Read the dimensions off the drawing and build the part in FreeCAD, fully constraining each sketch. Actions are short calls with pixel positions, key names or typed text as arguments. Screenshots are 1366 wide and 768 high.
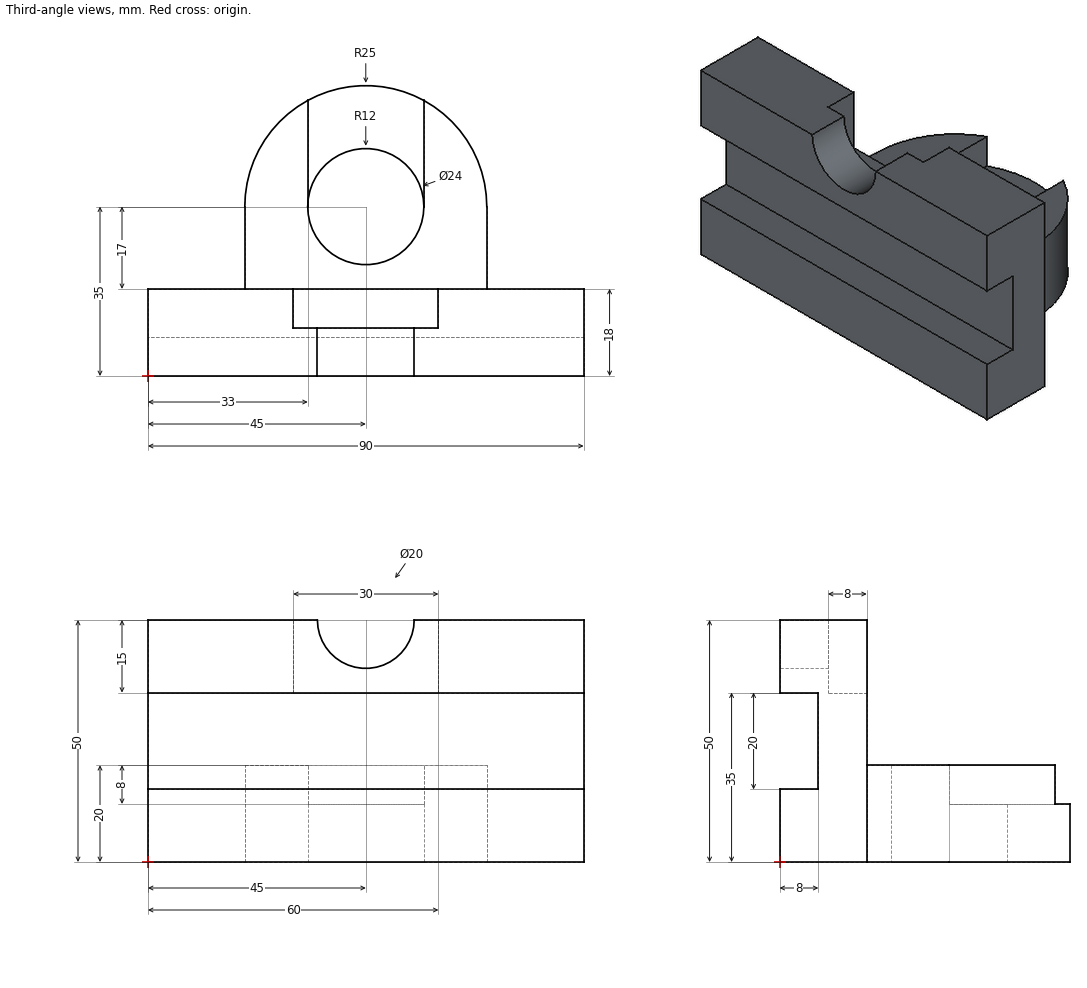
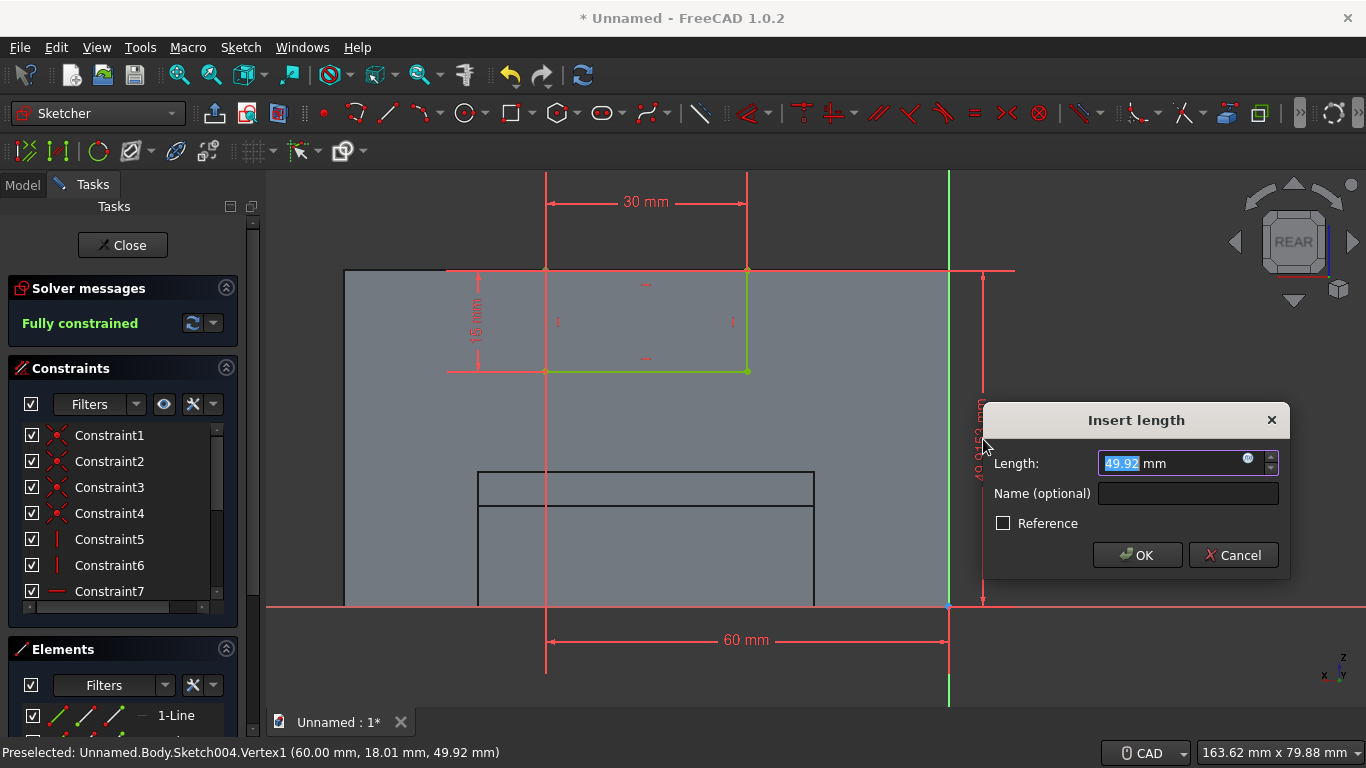
text(50)
key(Return)
key(Escape)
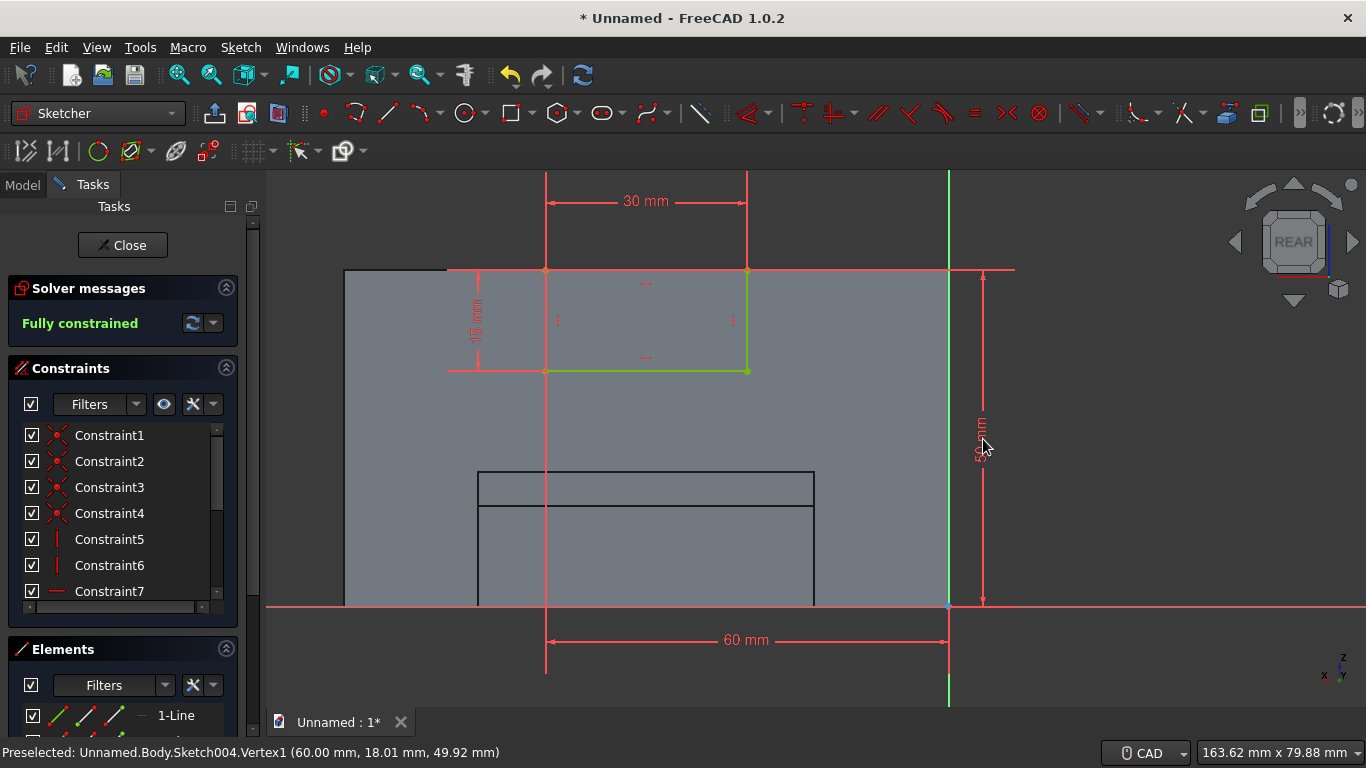
click(123, 245)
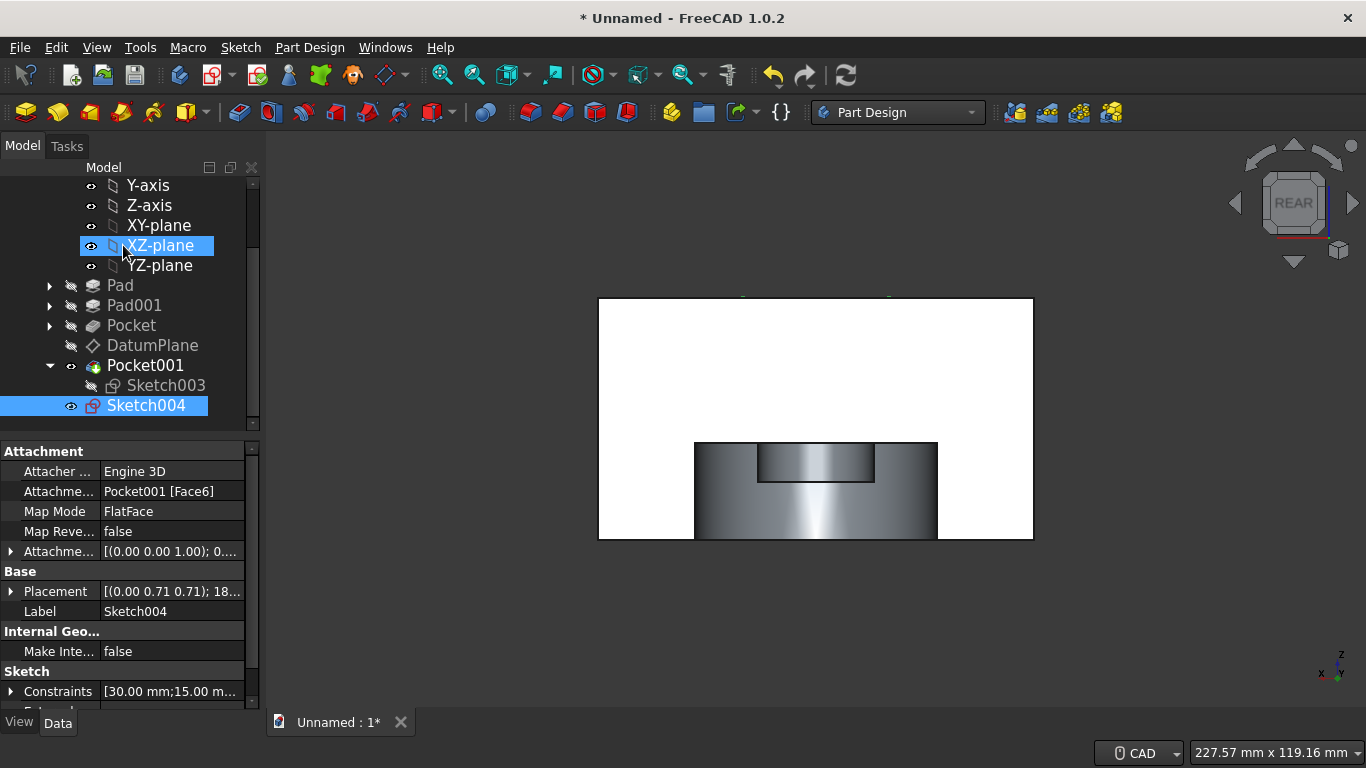
click(240, 112)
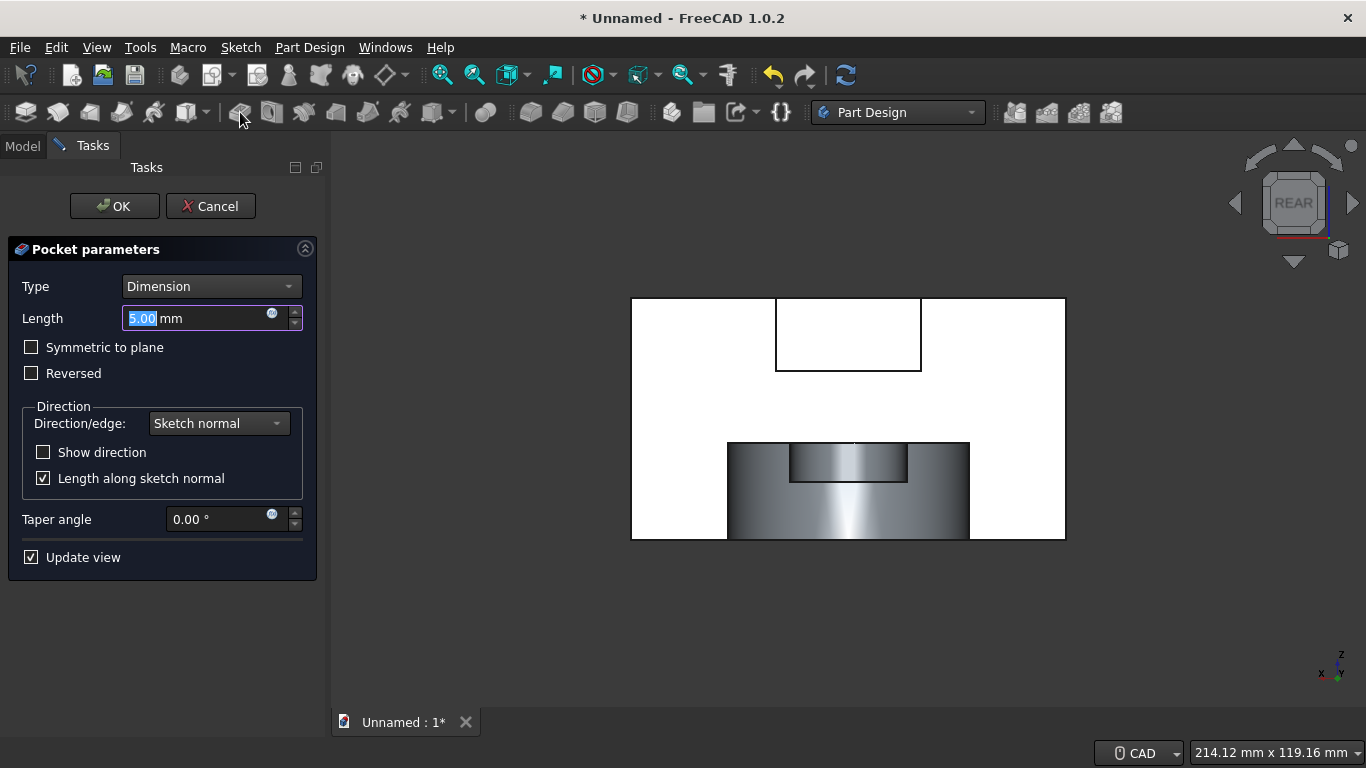
text(8)
key(Tab)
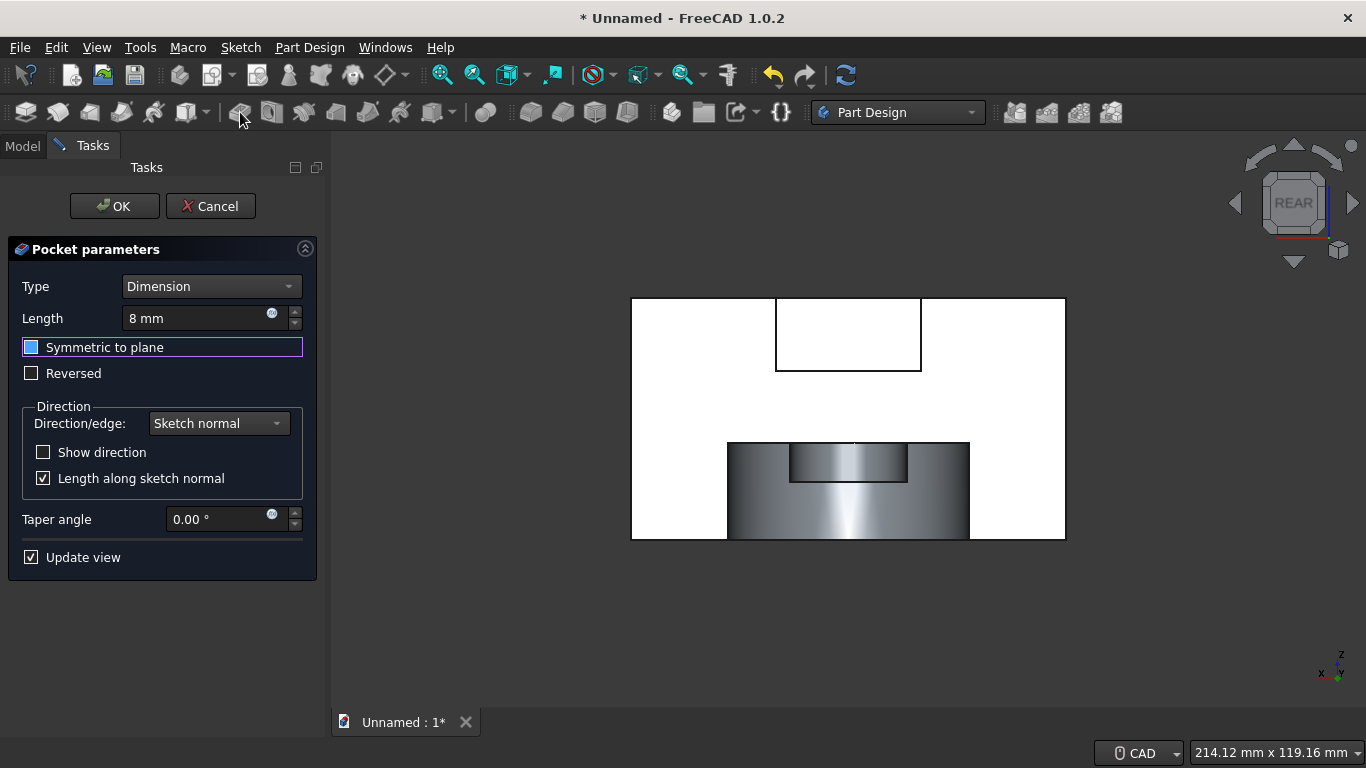
click(115, 206)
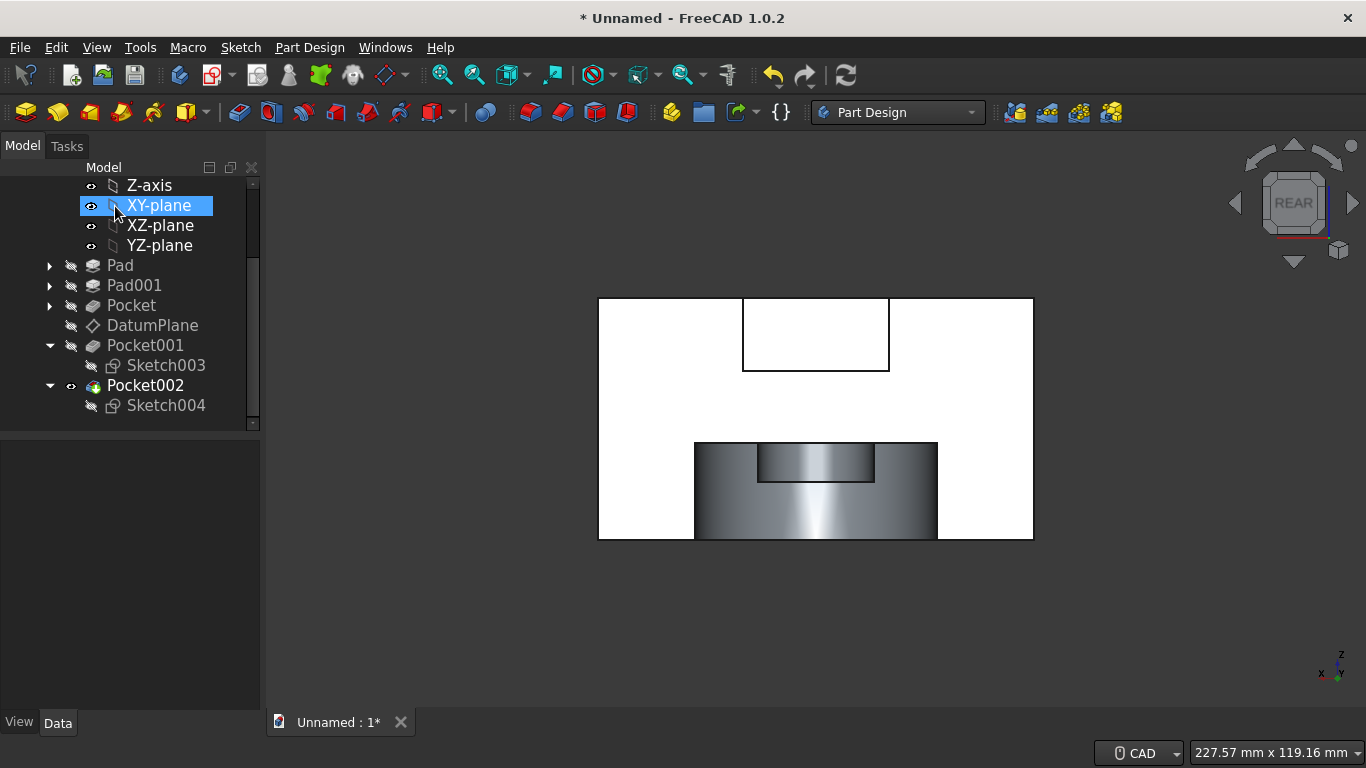
click(444, 76)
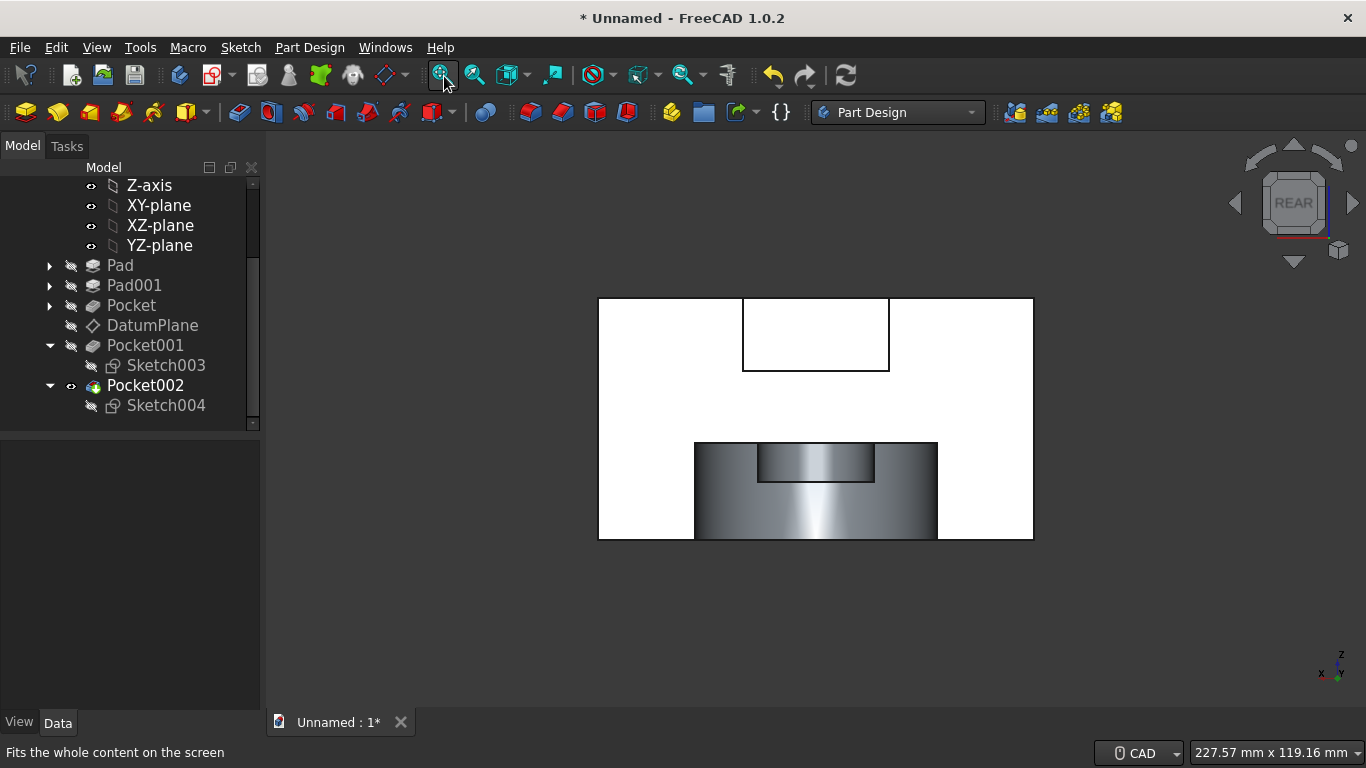
click(795, 333)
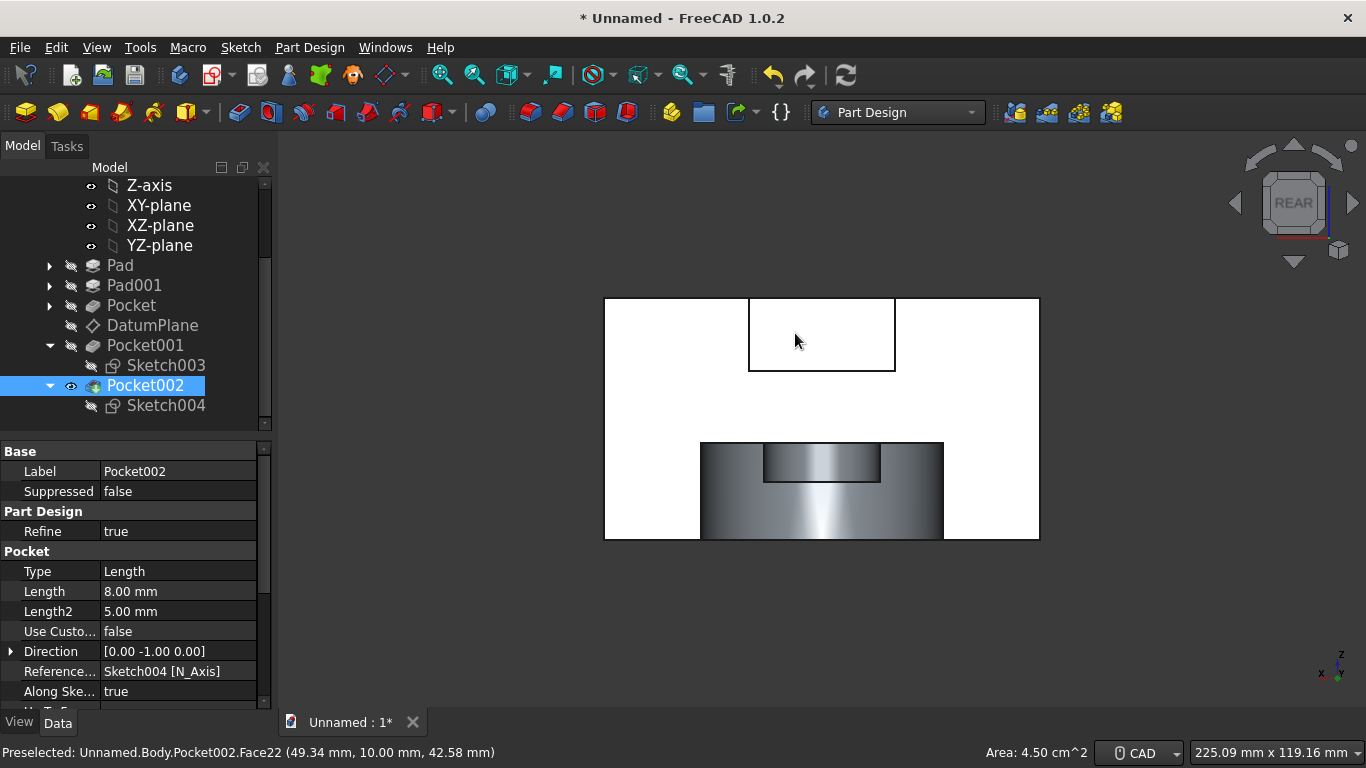
click(212, 76)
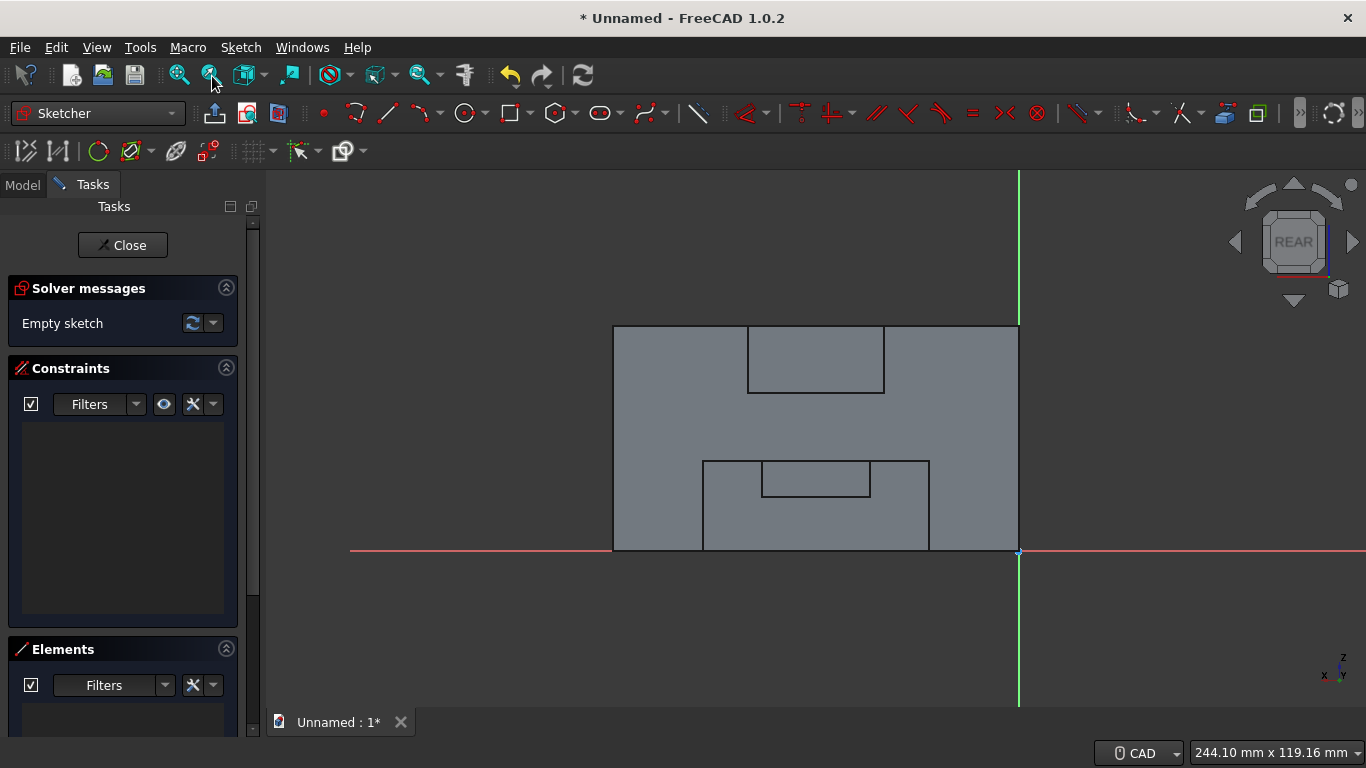
key(q)
key(s)